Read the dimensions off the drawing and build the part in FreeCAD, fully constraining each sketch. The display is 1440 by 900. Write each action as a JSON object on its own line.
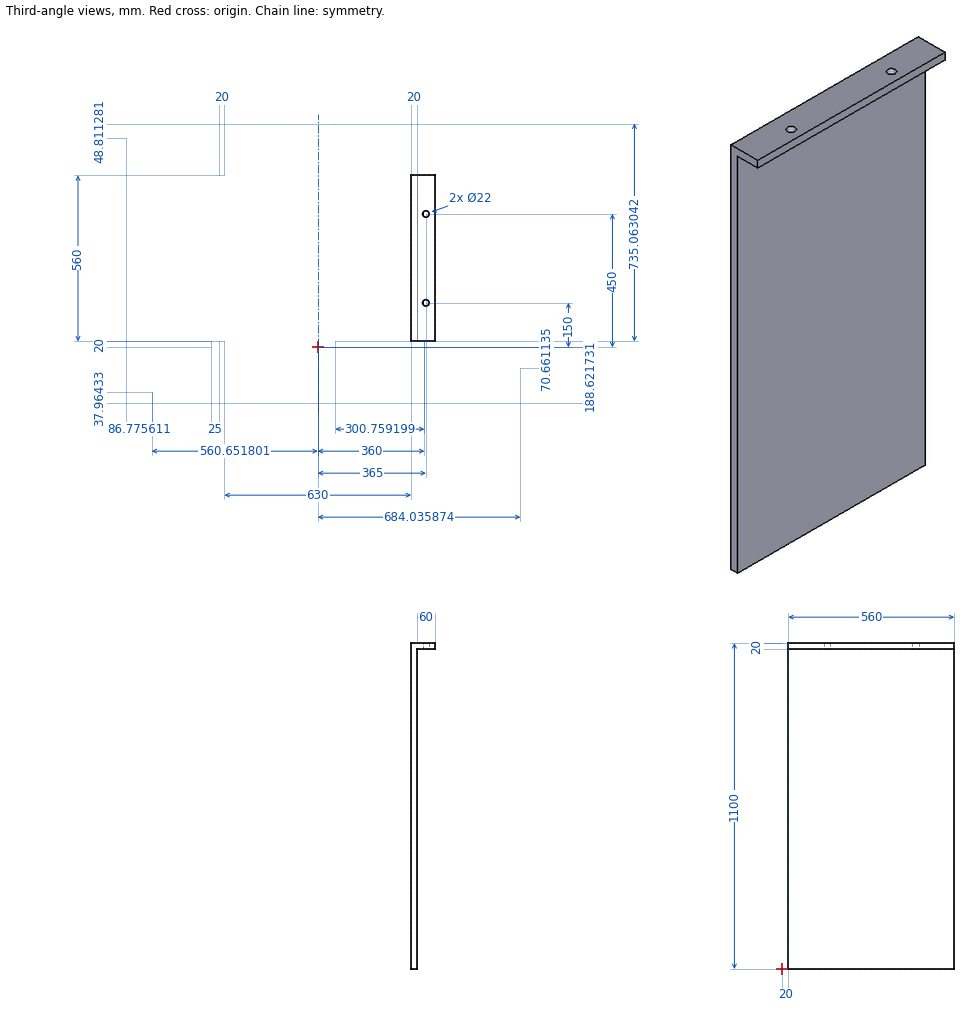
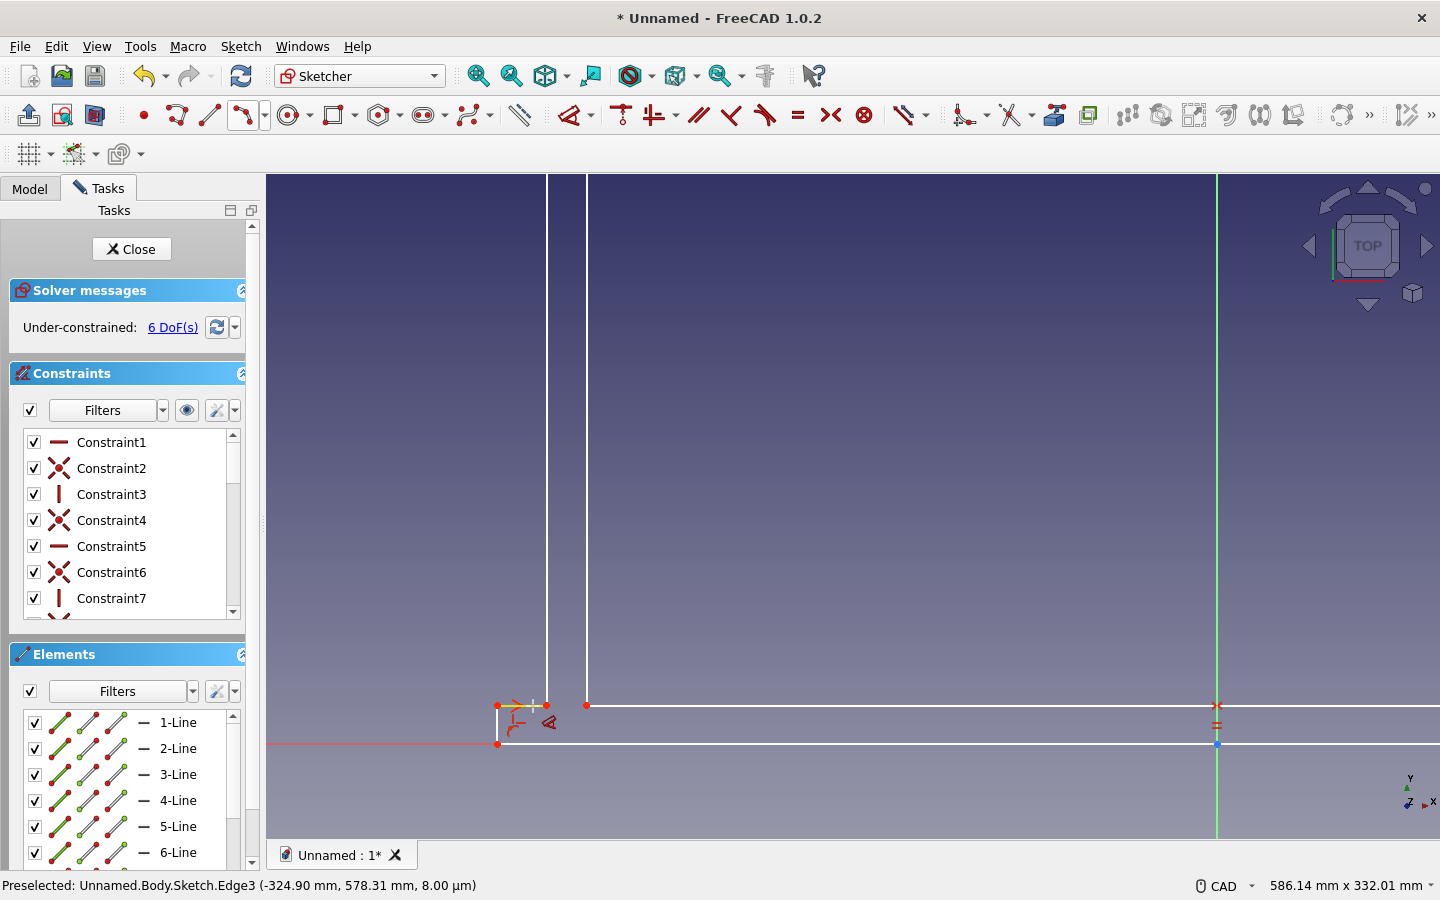
{"action": "left_click", "coordinate": [532, 706]}
{"action": "left_click", "coordinate": [522, 672]}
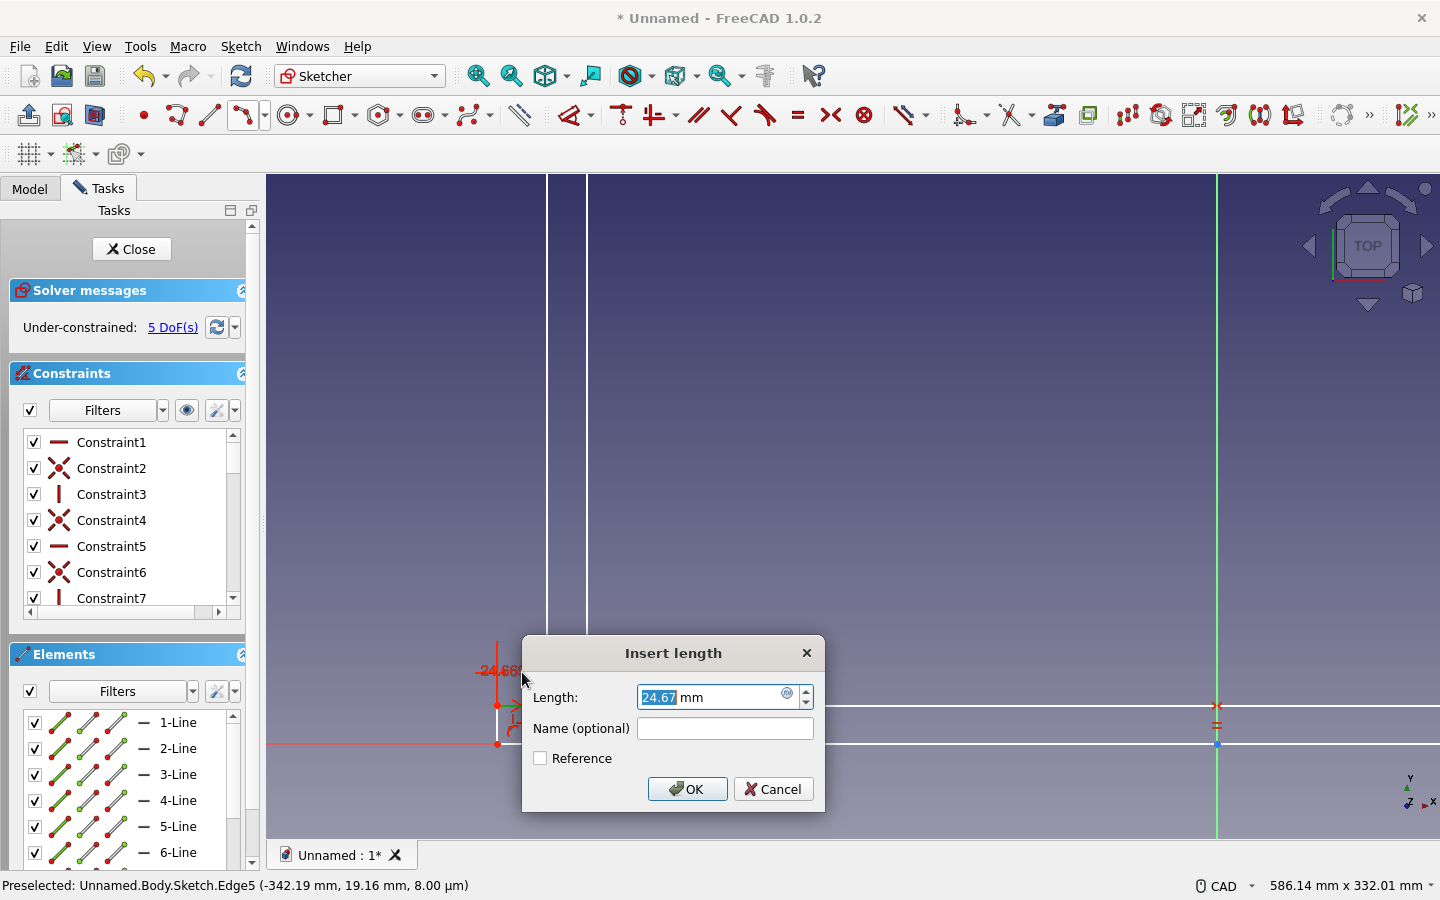
{"action": "type", "text": "25"}
{"action": "key", "text": "Return"}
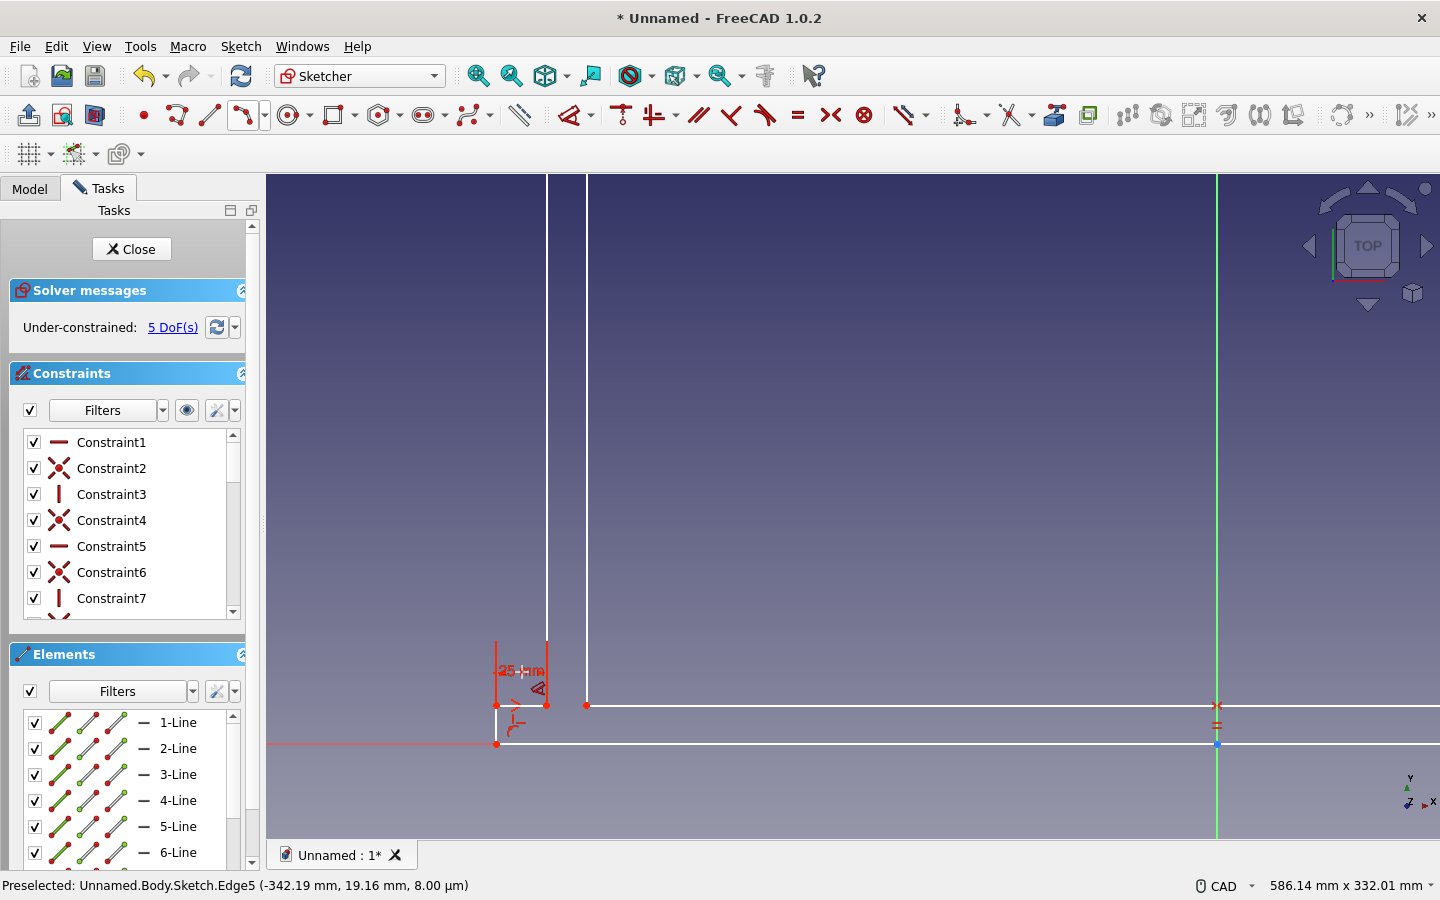
{"action": "left_click", "coordinate": [496, 717]}
{"action": "left_click", "coordinate": [462, 725]}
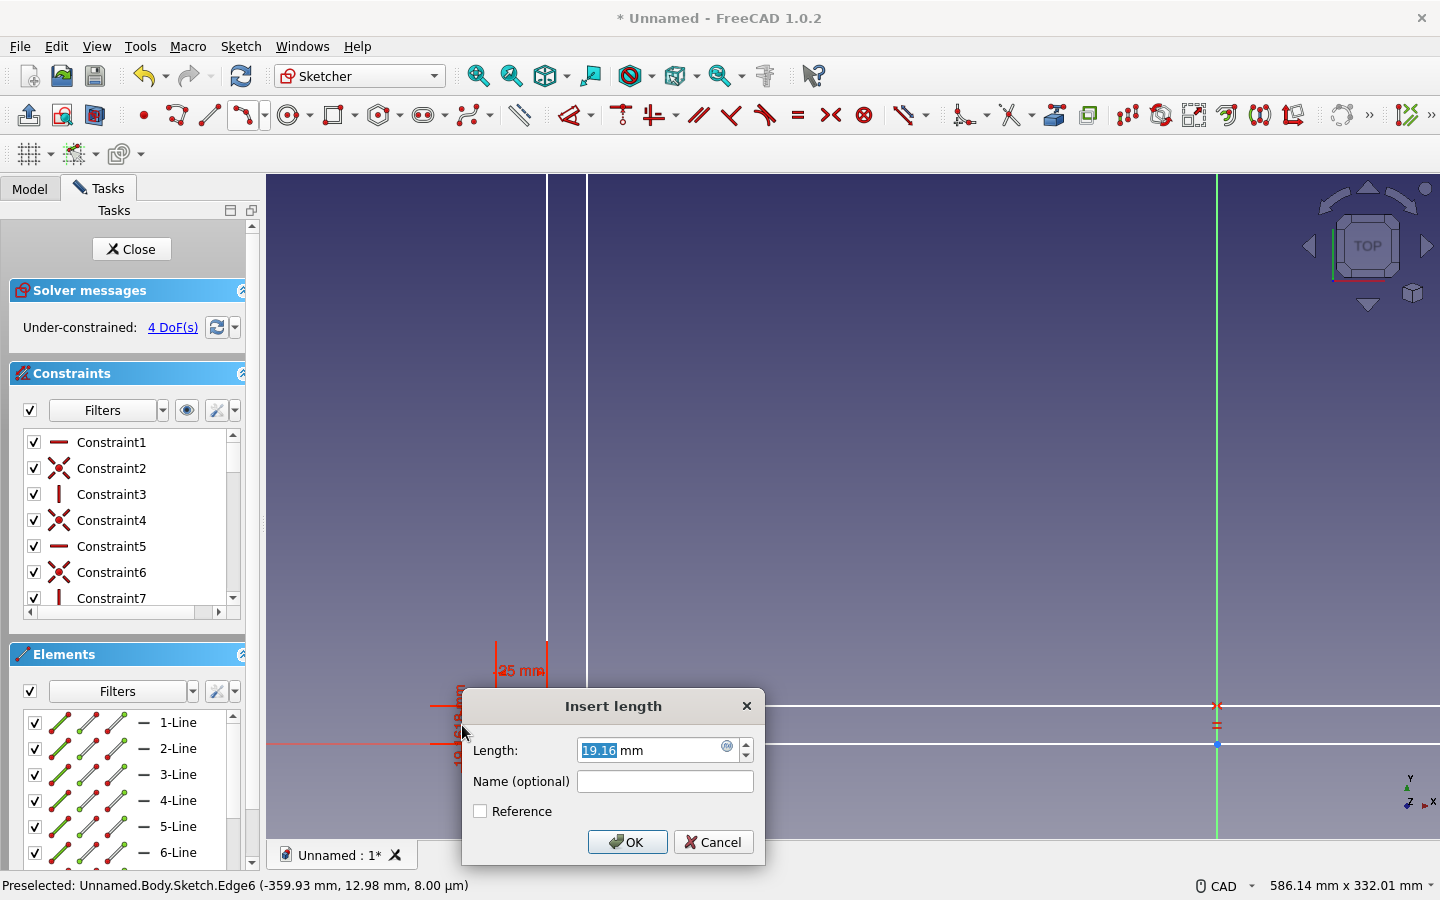
{"action": "type", "text": "20"}
{"action": "key", "text": "Return"}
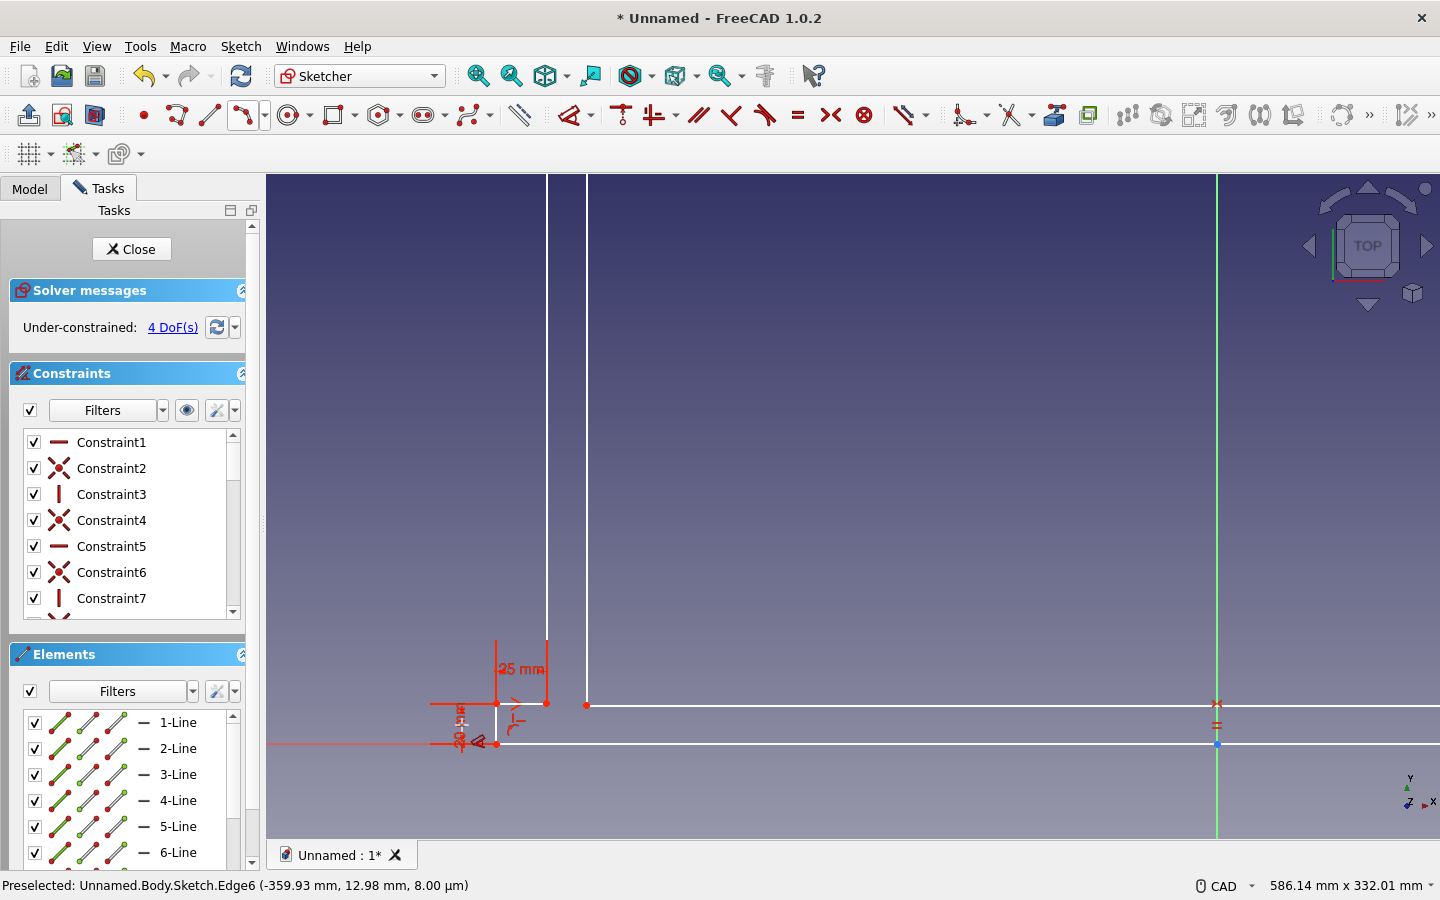
{"action": "scroll", "coordinate": [533, 706], "scroll_direction": "down", "scroll_amount": 5}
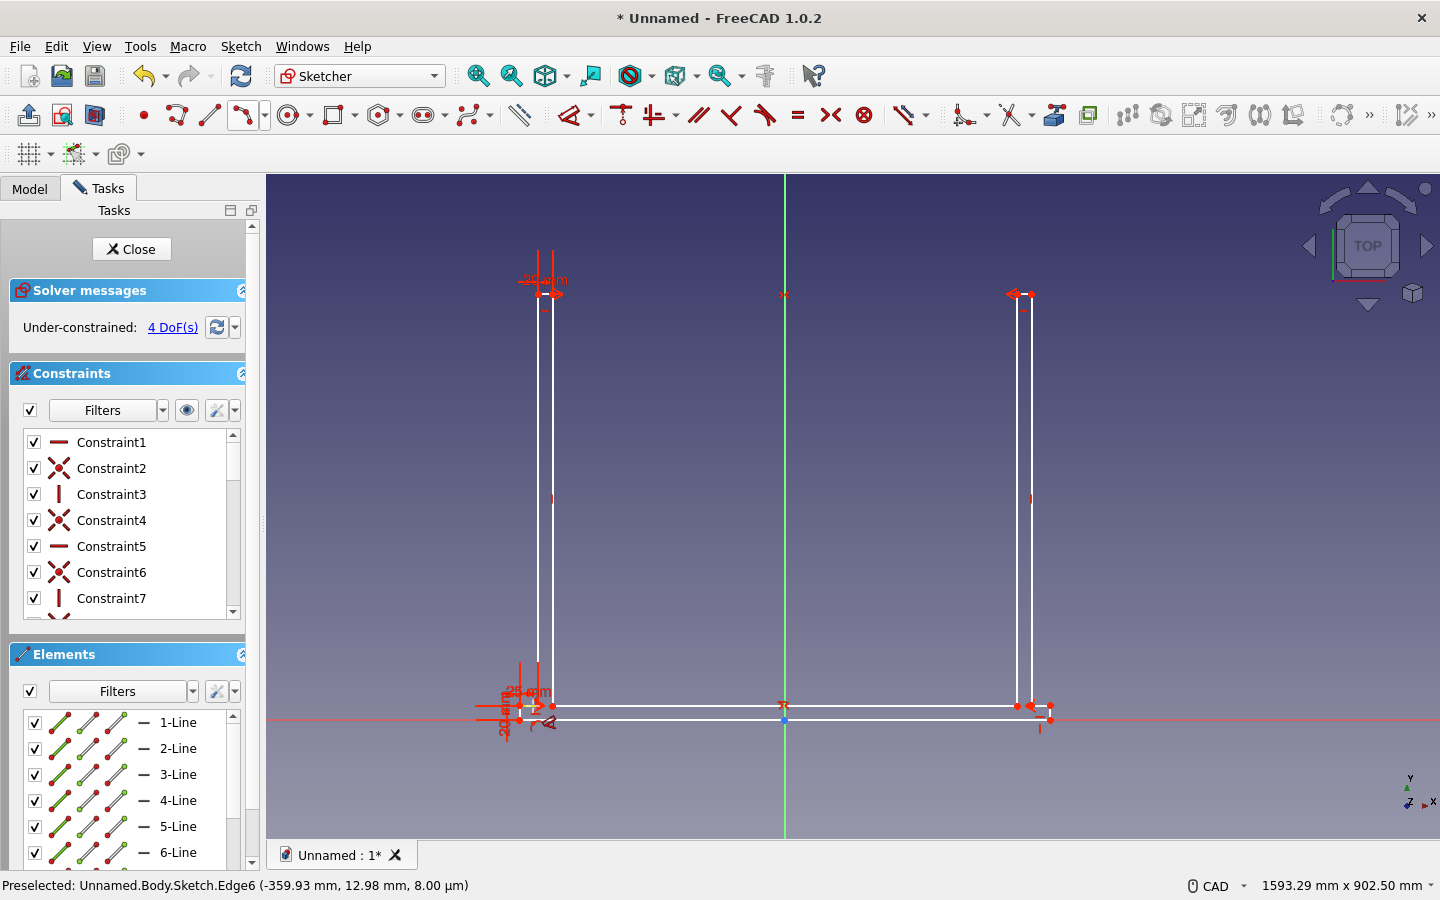
{"action": "scroll", "coordinate": [1027, 294], "scroll_direction": "up", "scroll_amount": 6}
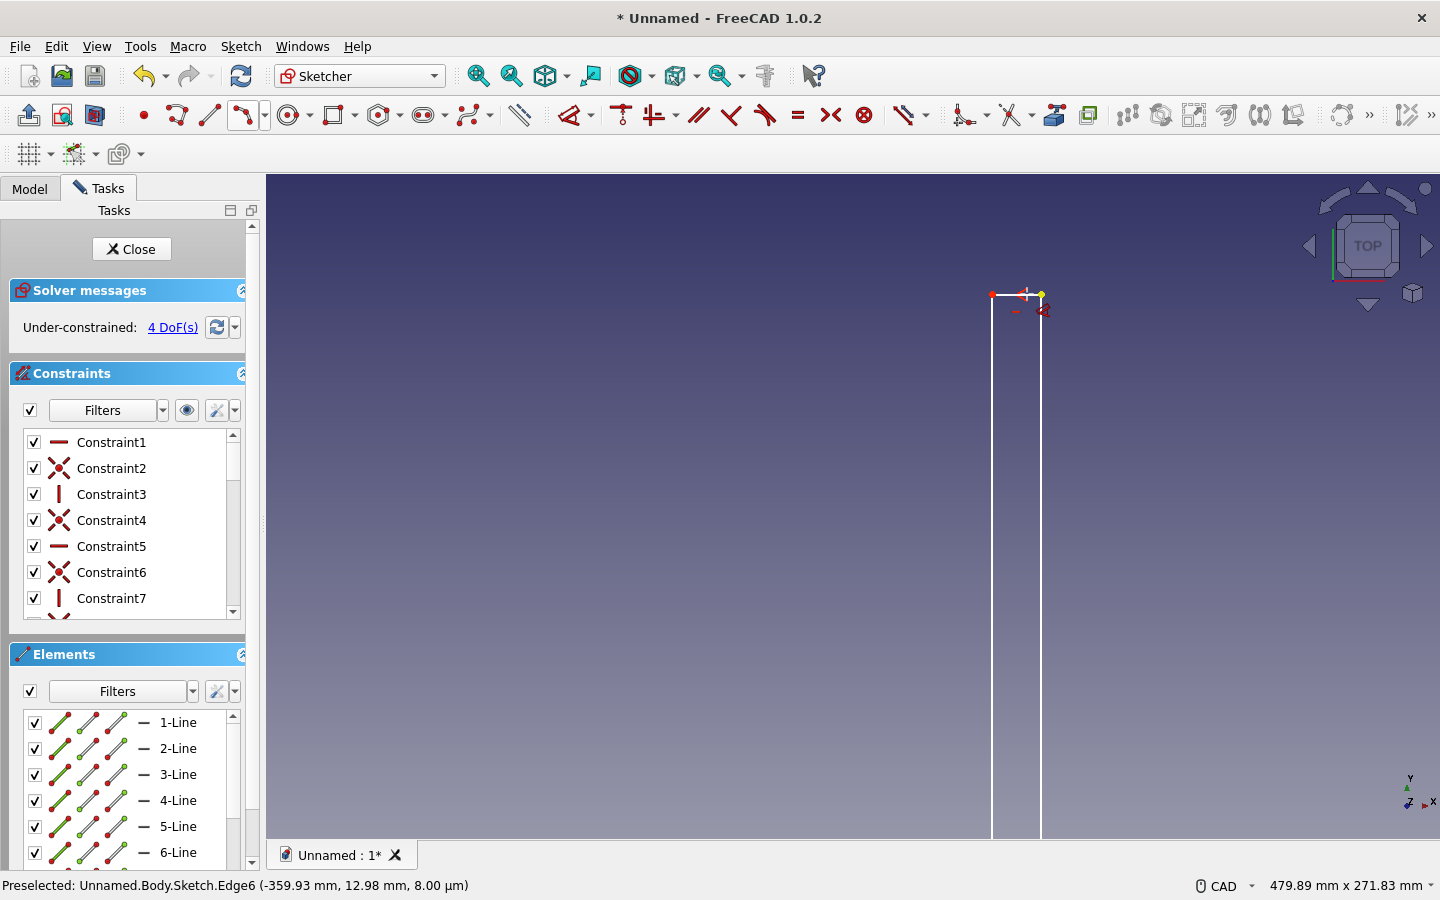
{"action": "left_click", "coordinate": [1026, 295]}
{"action": "left_click", "coordinate": [1017, 261]}